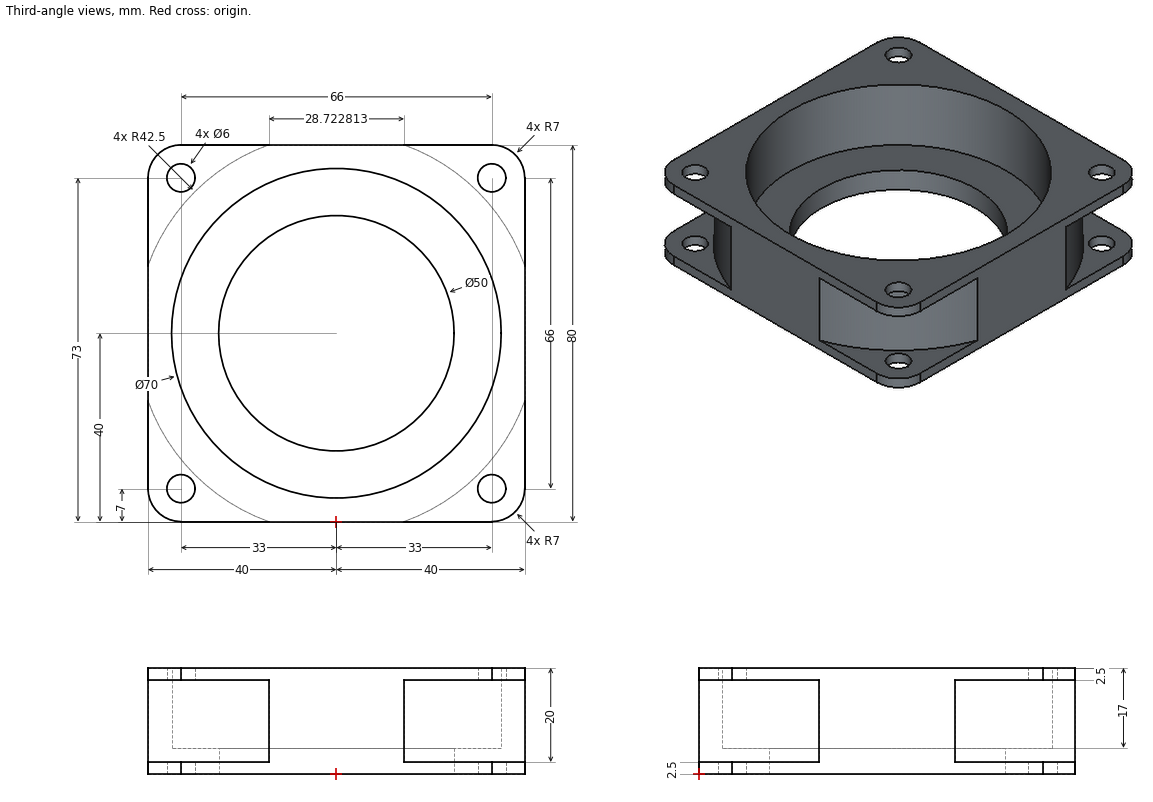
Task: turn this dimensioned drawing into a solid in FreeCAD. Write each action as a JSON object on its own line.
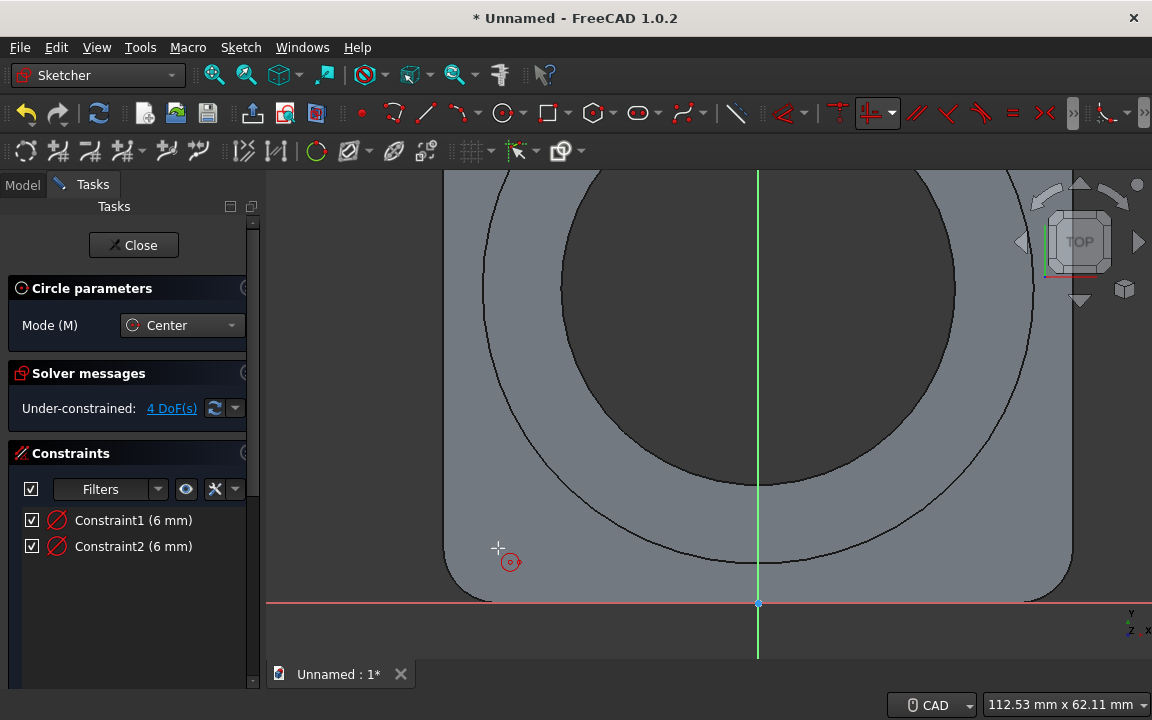
{"action": "left_click", "coordinate": [498, 548]}
{"action": "mouse_move", "coordinate": [515, 531]}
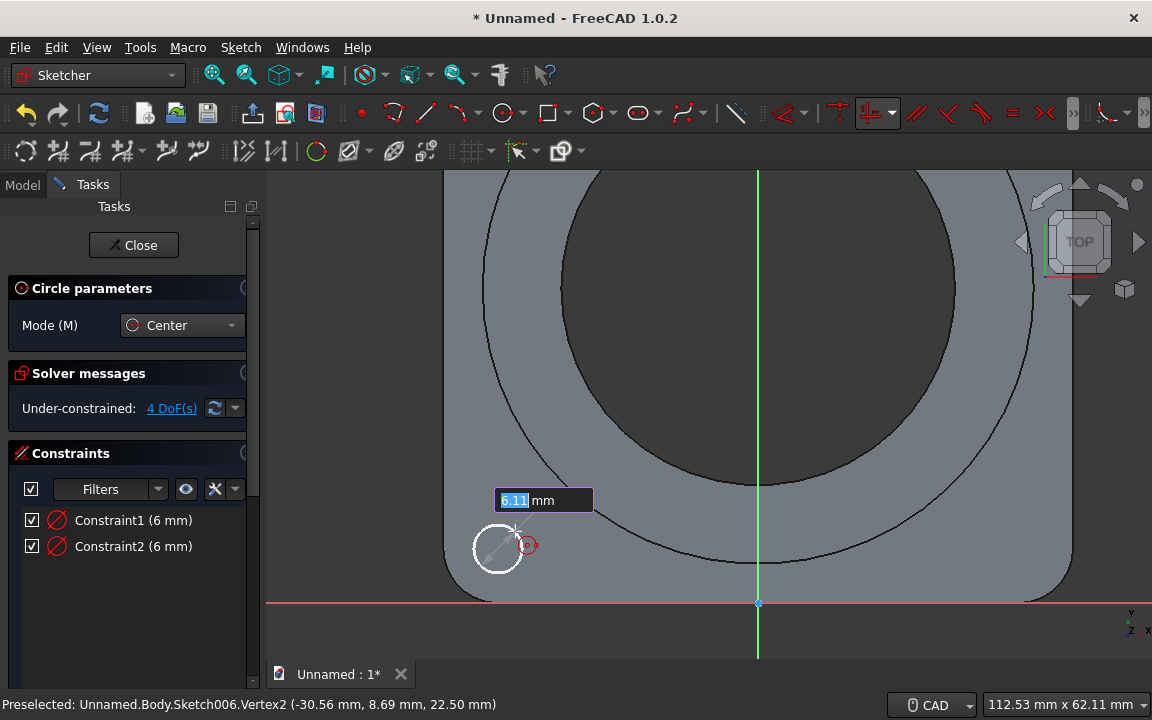
{"action": "type", "text": "6"}
{"action": "key", "text": "Return"}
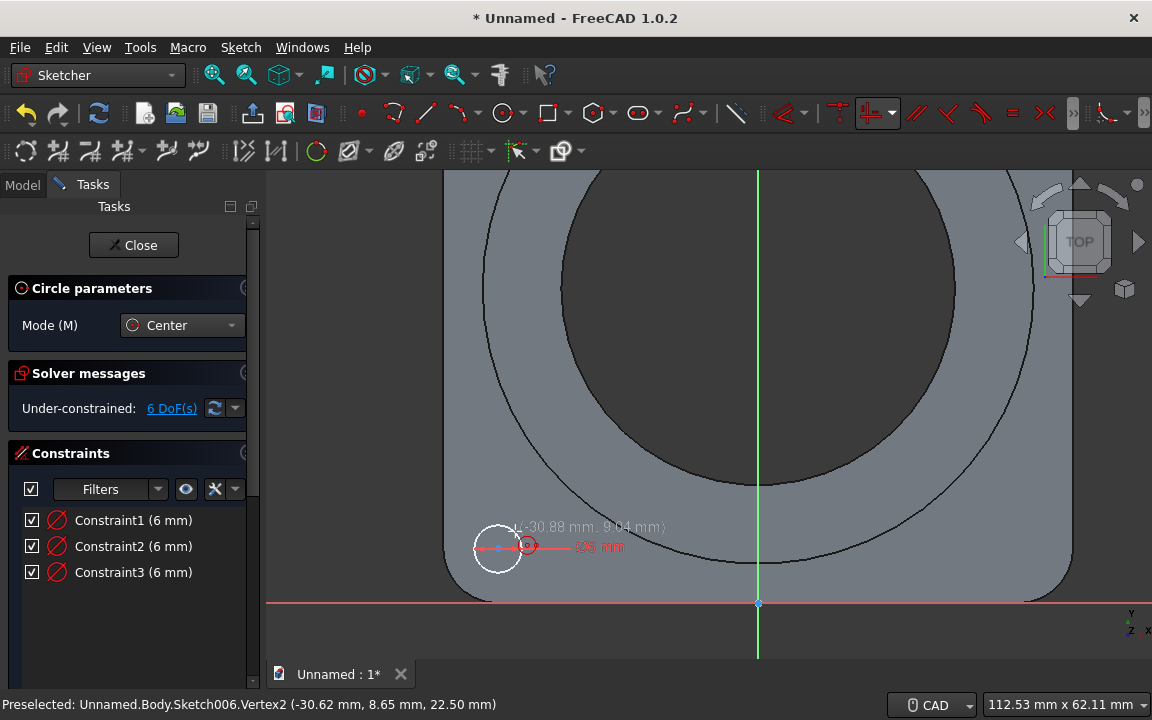
{"action": "scroll", "coordinate": [497, 549], "scroll_direction": "down", "scroll_amount": 3}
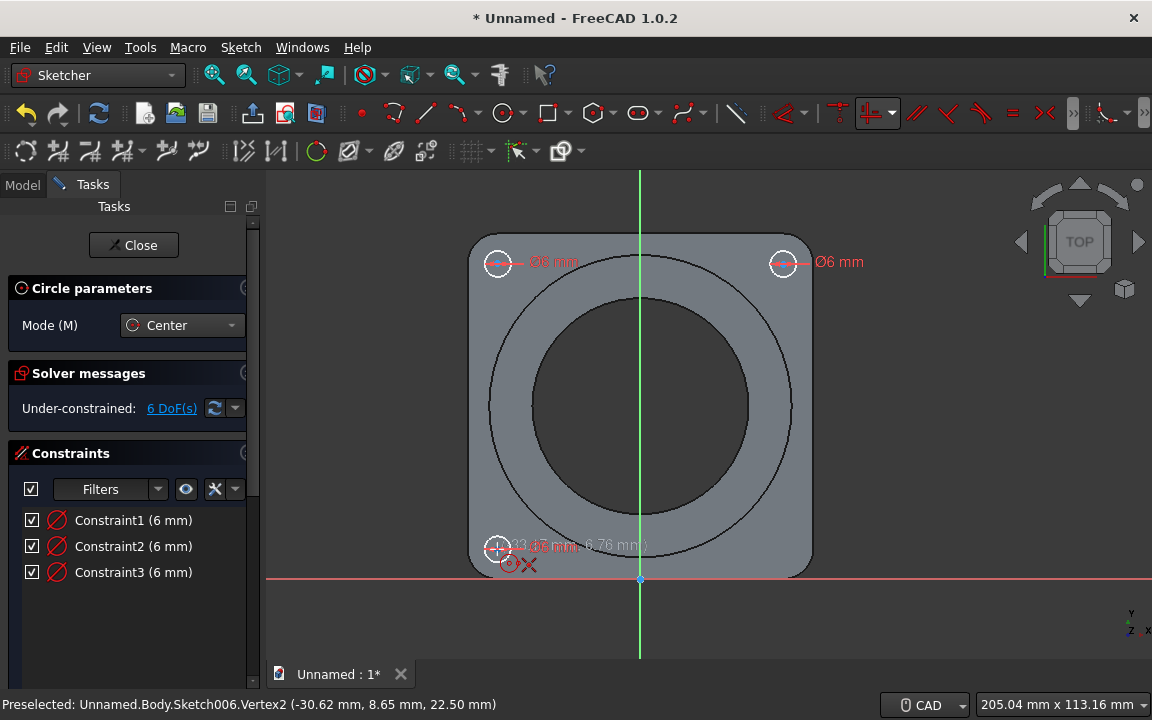
{"action": "scroll", "coordinate": [783, 549], "scroll_direction": "up", "scroll_amount": 3}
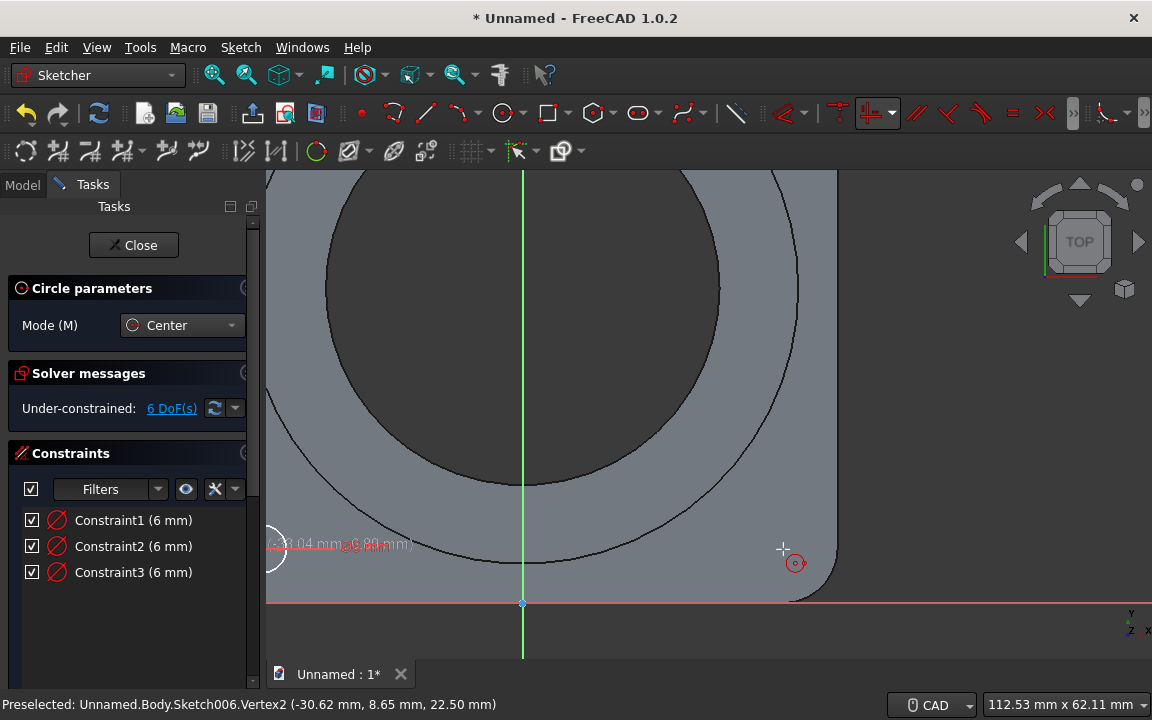
{"action": "left_click", "coordinate": [783, 548]}
{"action": "mouse_move", "coordinate": [799, 531]}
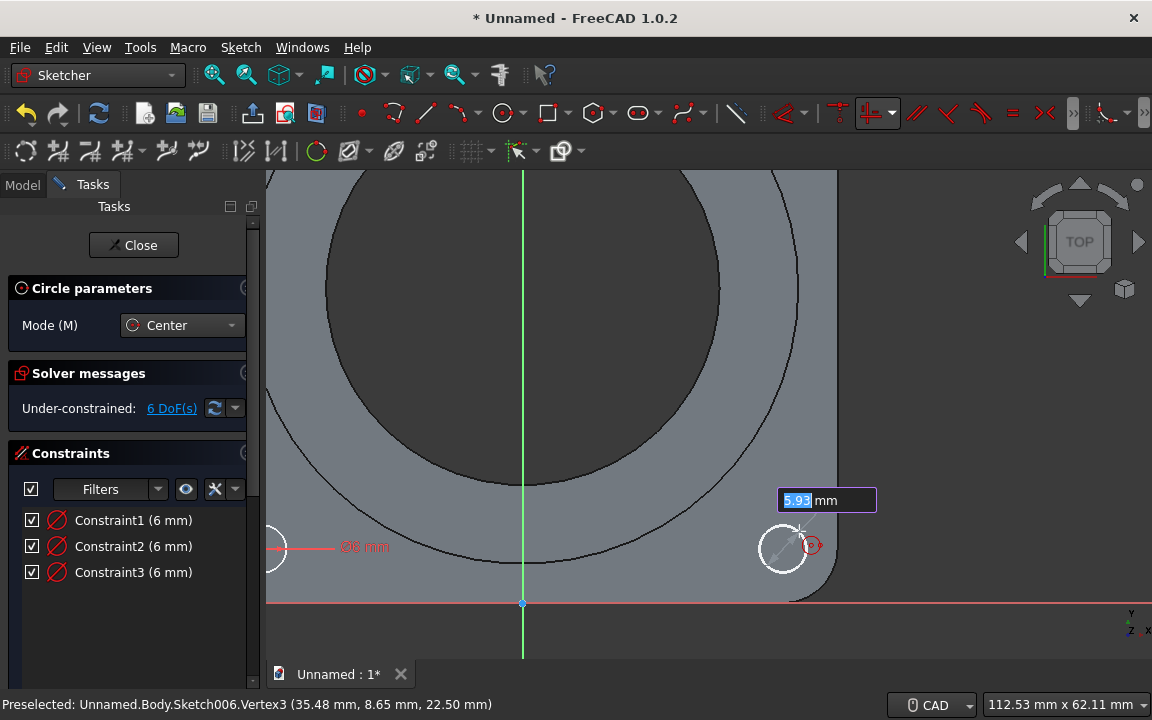
{"action": "type", "text": "6"}
{"action": "key", "text": "Return"}
{"action": "key", "text": "Escape"}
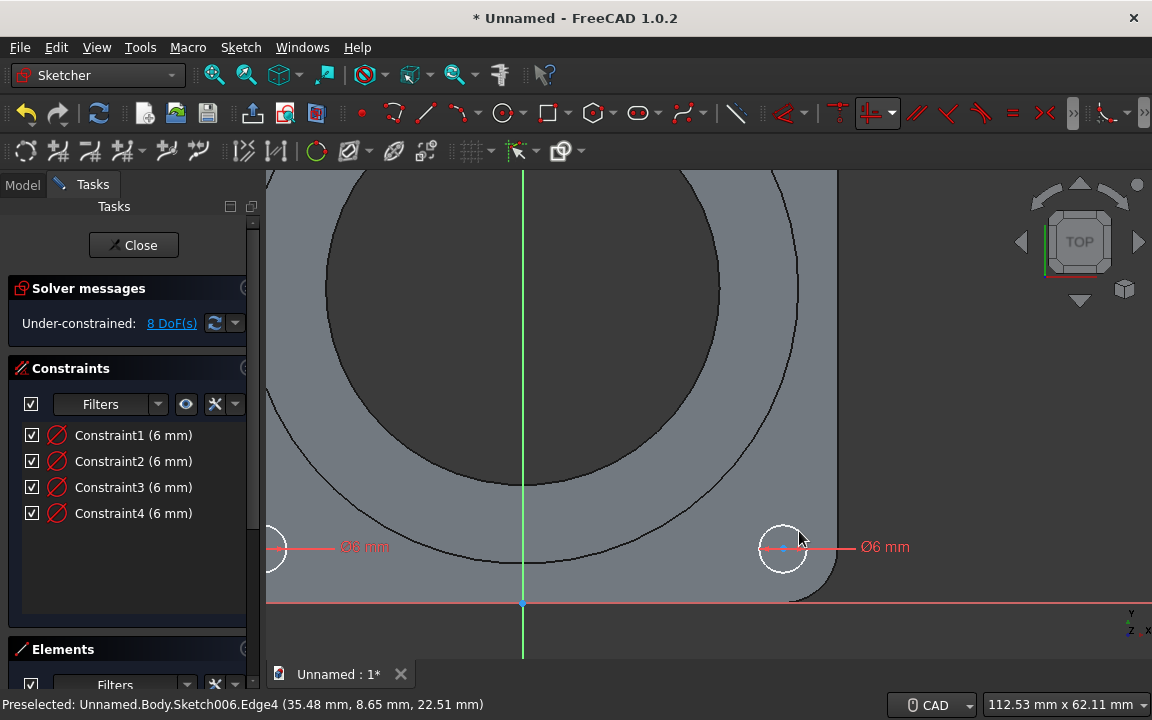
{"action": "scroll", "coordinate": [784, 549], "scroll_direction": "down", "scroll_amount": 3}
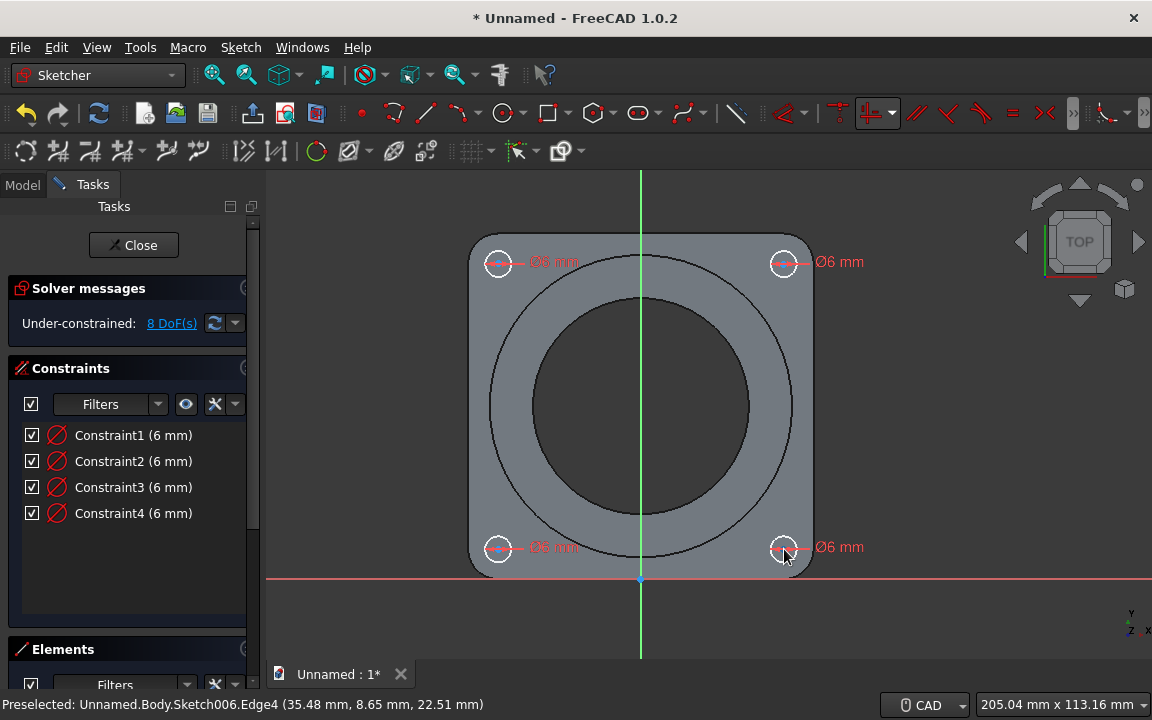
{"action": "left_click", "coordinate": [498, 264]}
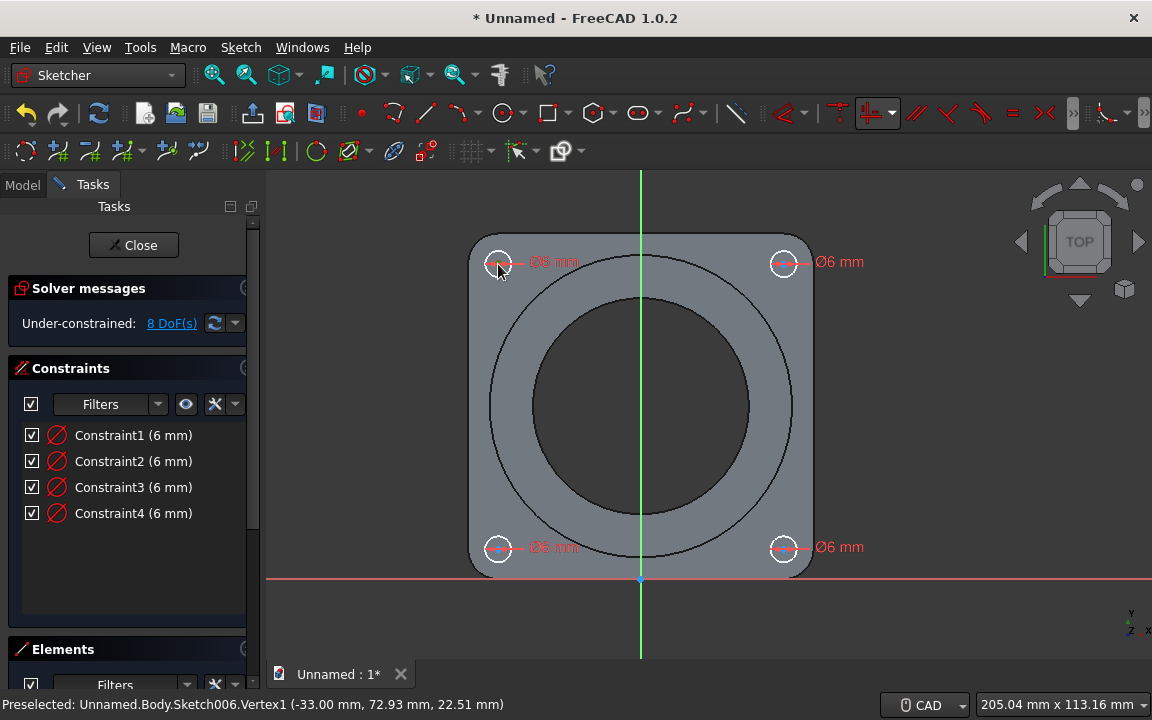
{"action": "left_click", "coordinate": [784, 264]}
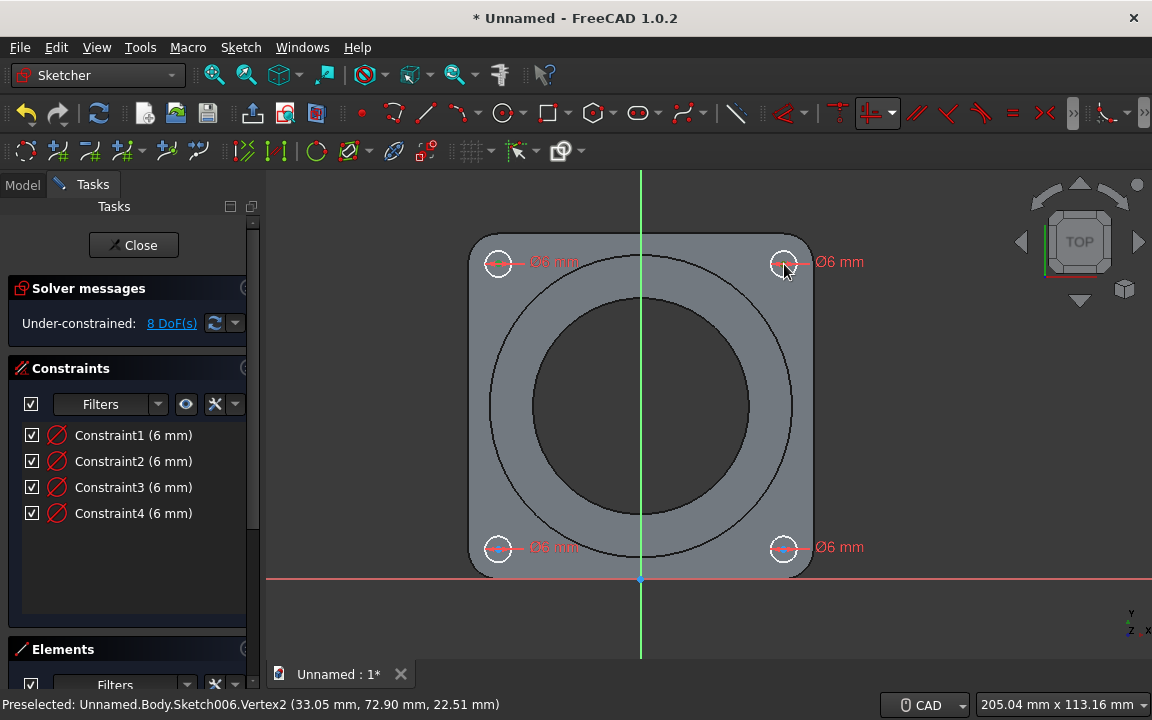
{"action": "key", "text": "h"}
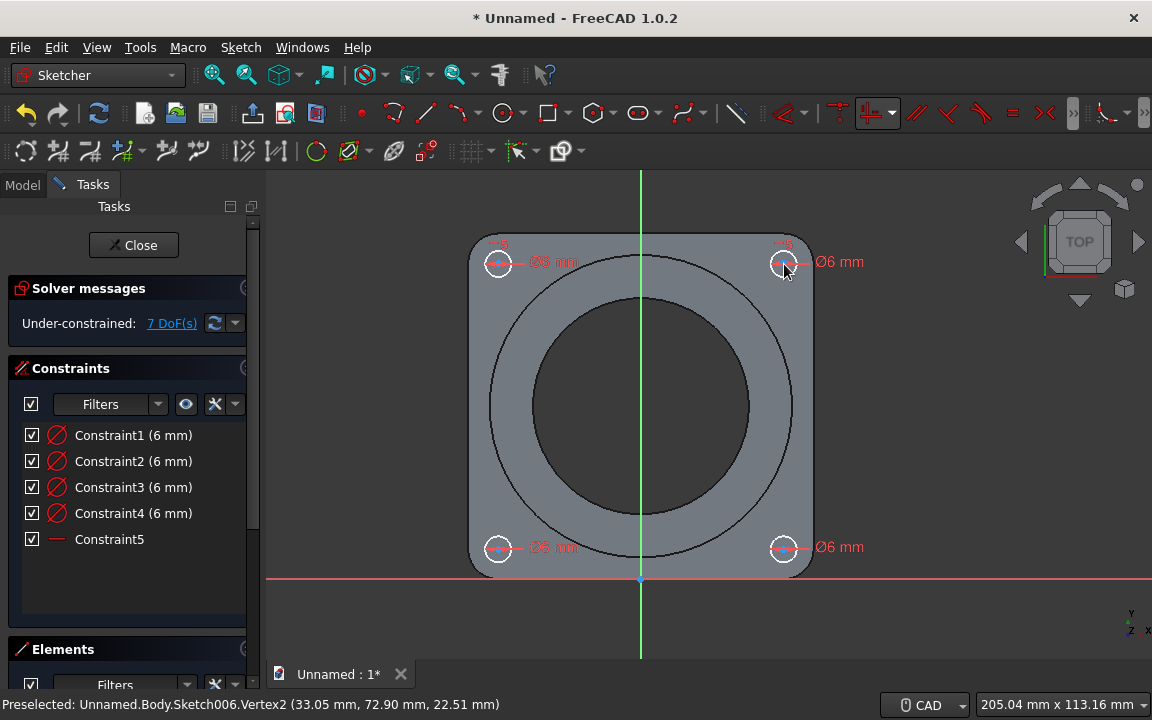
{"action": "left_click", "coordinate": [498, 264]}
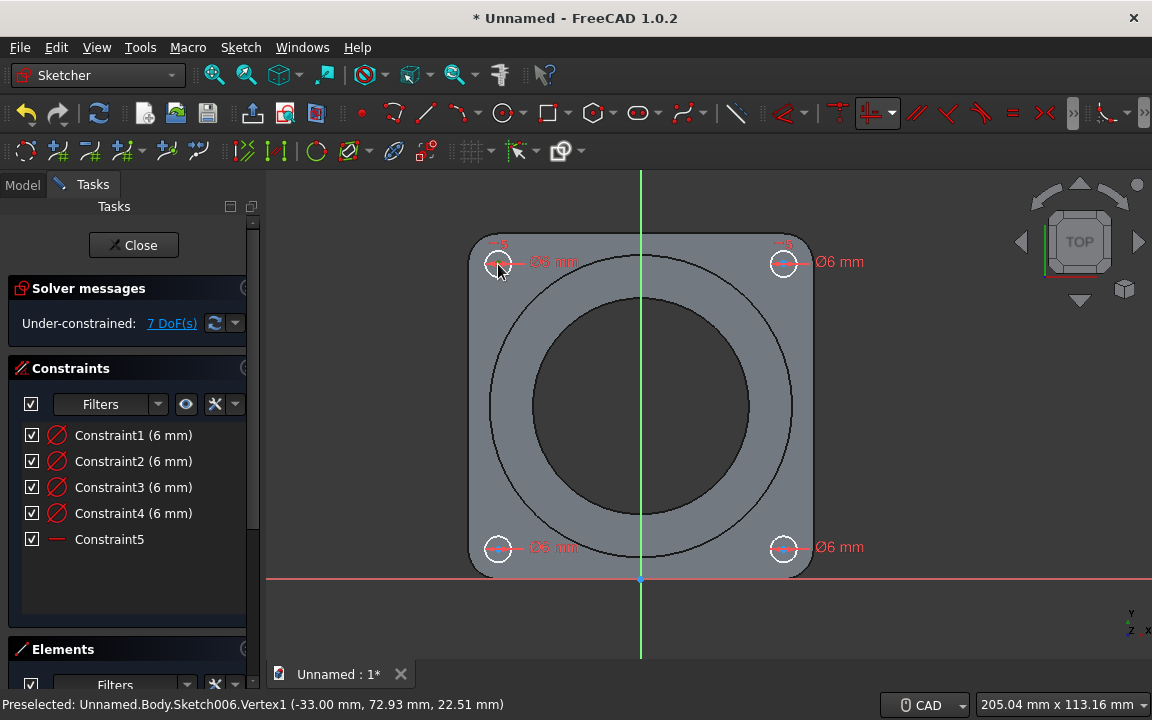
{"action": "left_click", "coordinate": [498, 549]}